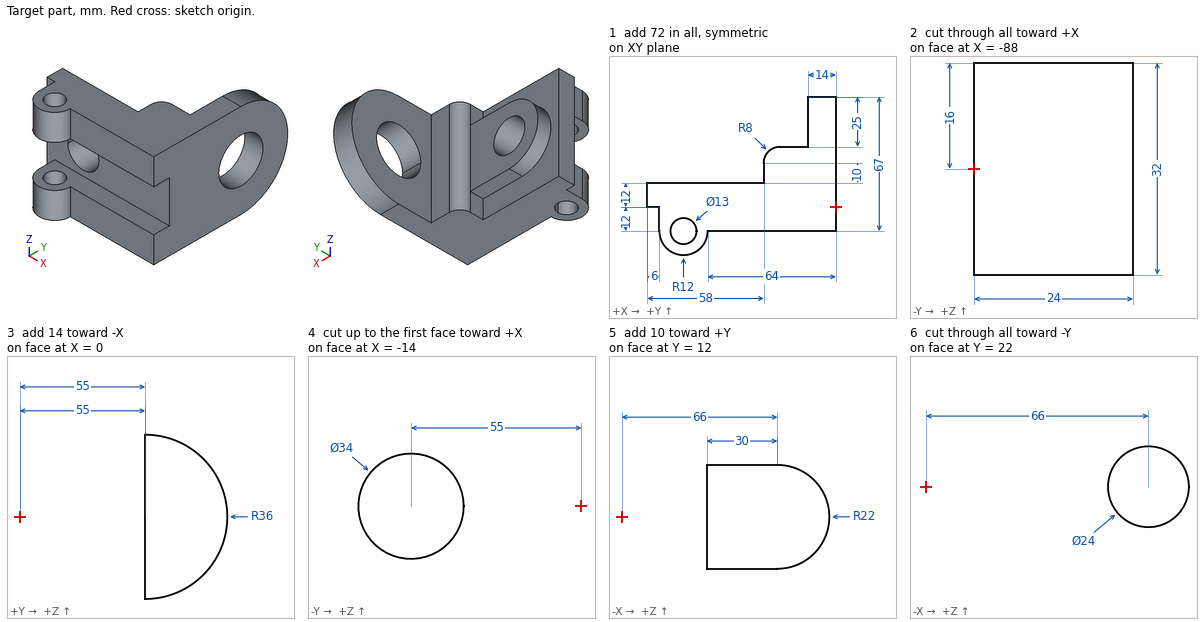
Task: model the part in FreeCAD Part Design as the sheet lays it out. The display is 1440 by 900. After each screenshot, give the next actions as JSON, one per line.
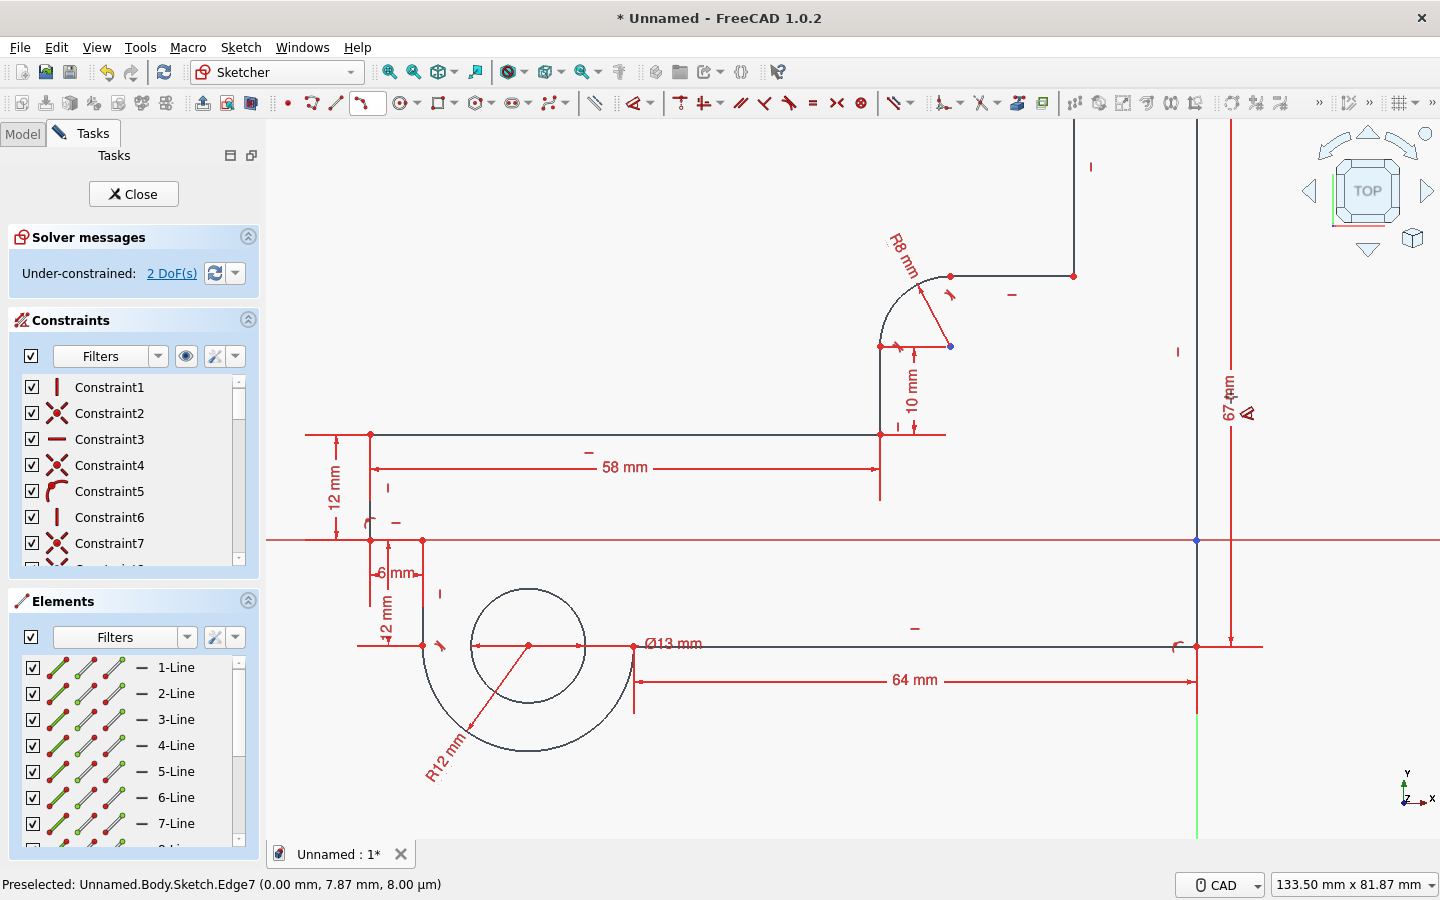
{"action": "scroll", "coordinate": [787, 632], "scroll_direction": "down", "scroll_amount": 2}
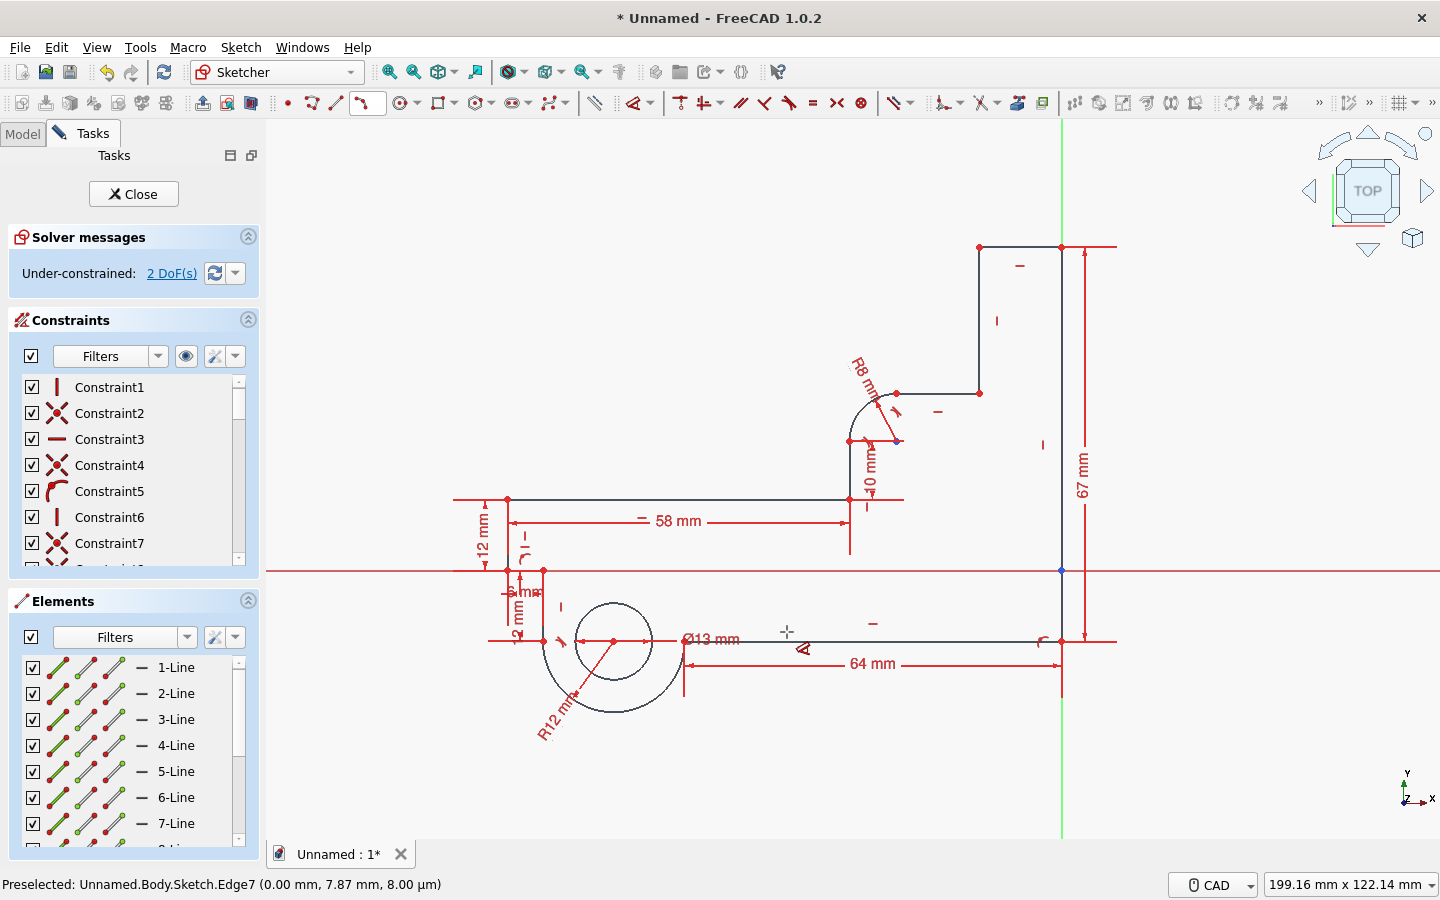
{"action": "left_click", "coordinate": [1037, 247]}
{"action": "left_click", "coordinate": [1021, 213]}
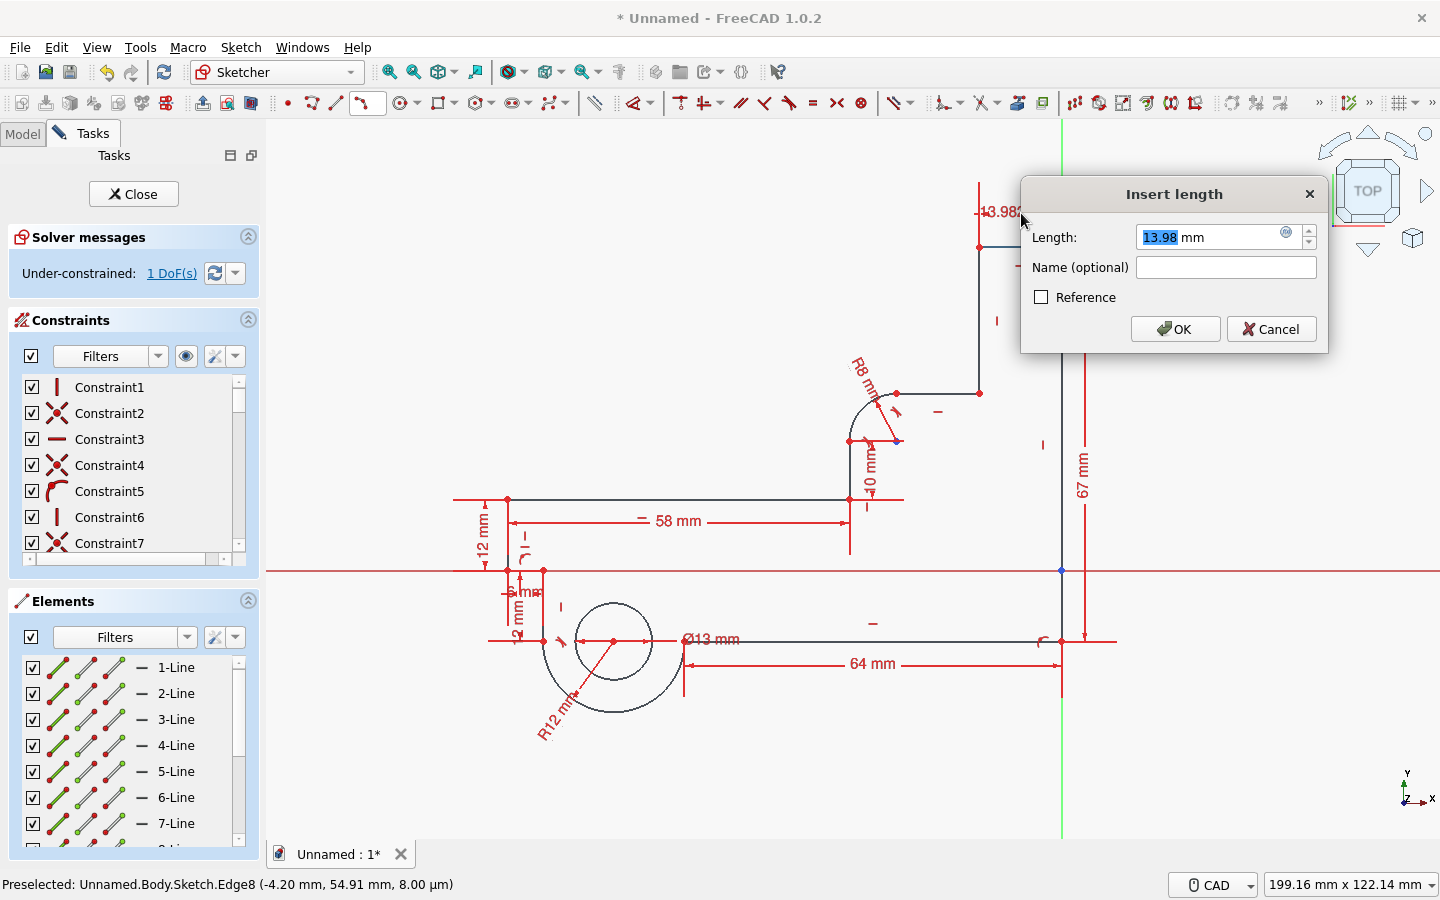
{"action": "type", "text": "14"}
{"action": "key", "text": "Return"}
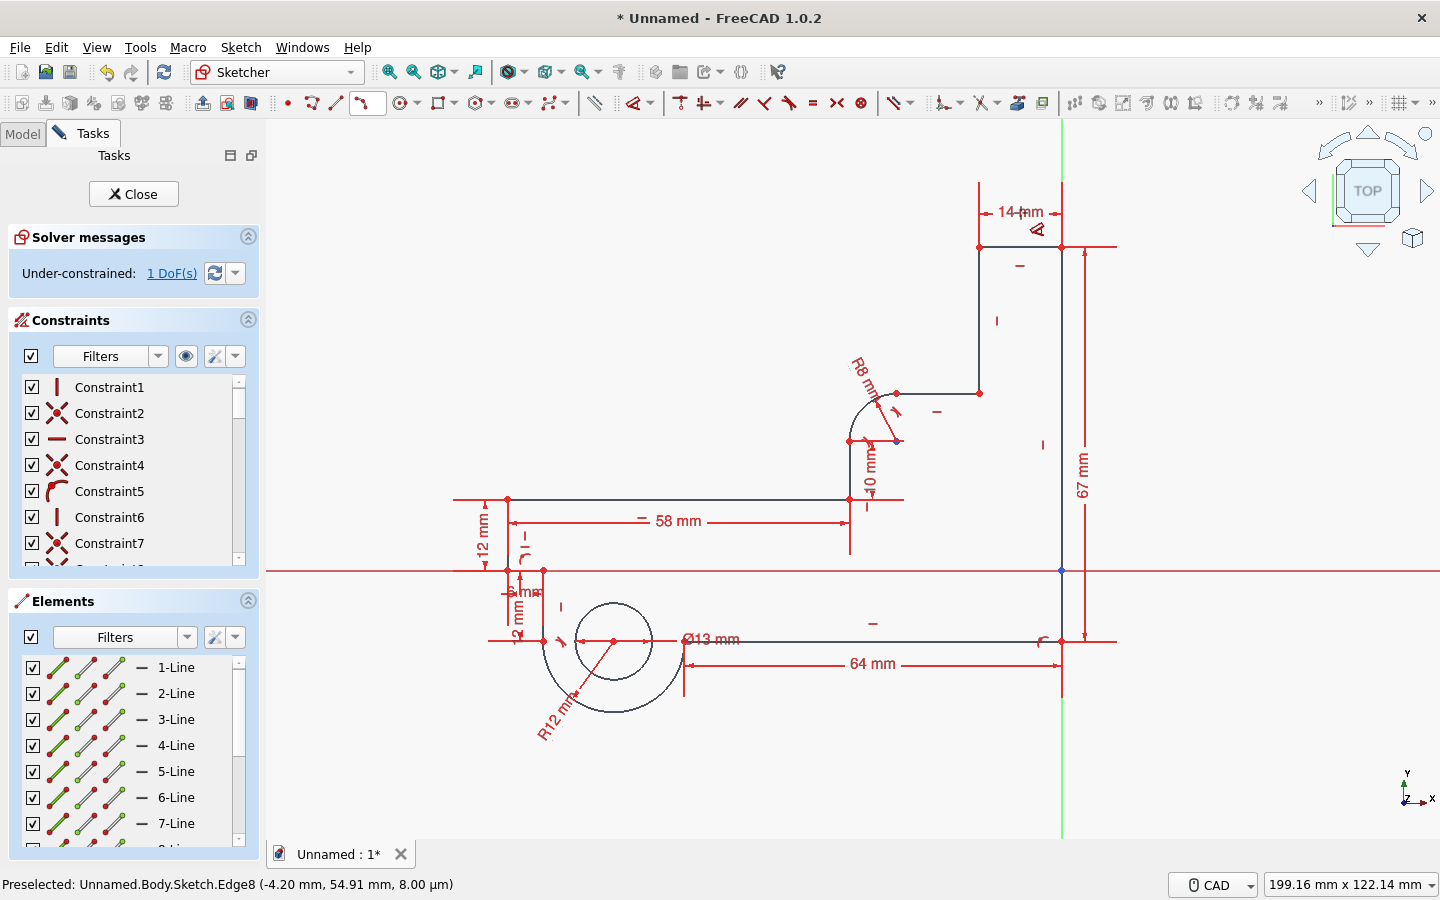
{"action": "left_click", "coordinate": [979, 291]}
{"action": "left_click", "coordinate": [1013, 320]}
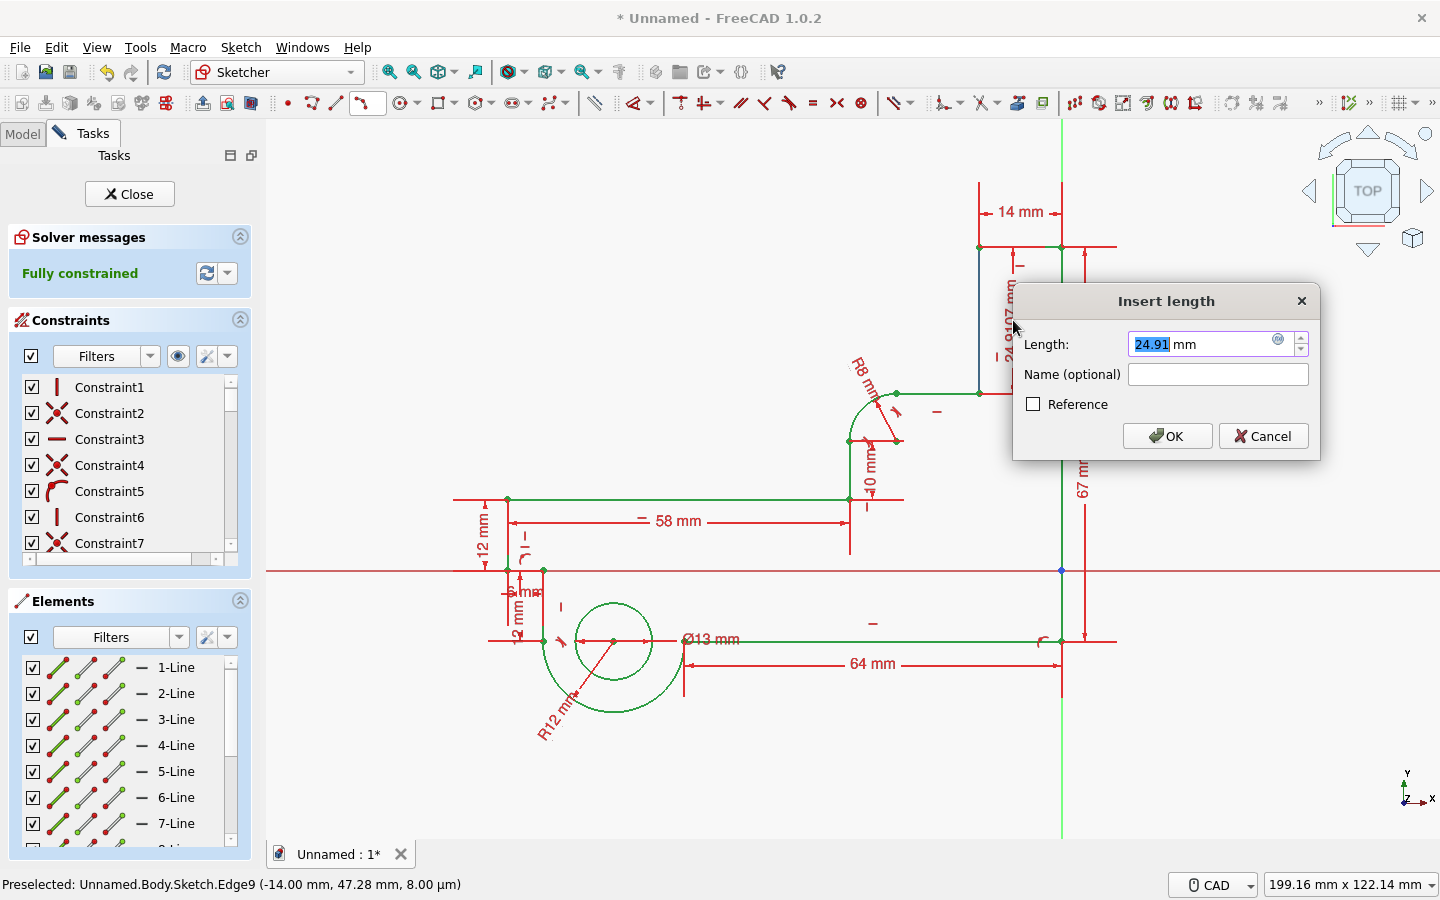
{"action": "type", "text": "25"}
{"action": "key", "text": "Return"}
{"action": "key", "text": "Escape"}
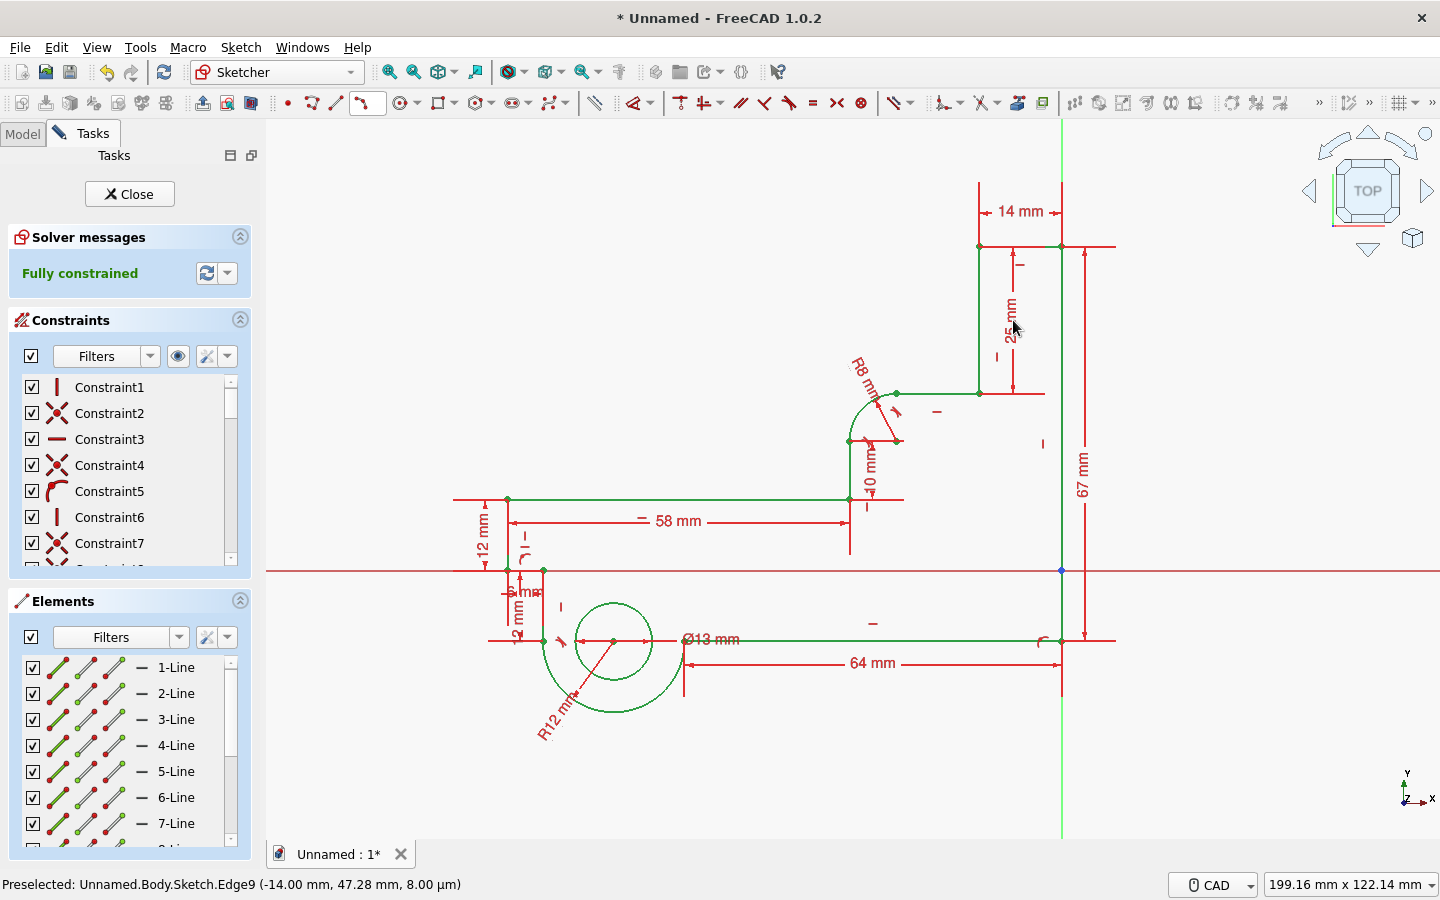
{"action": "left_click", "coordinate": [130, 194]}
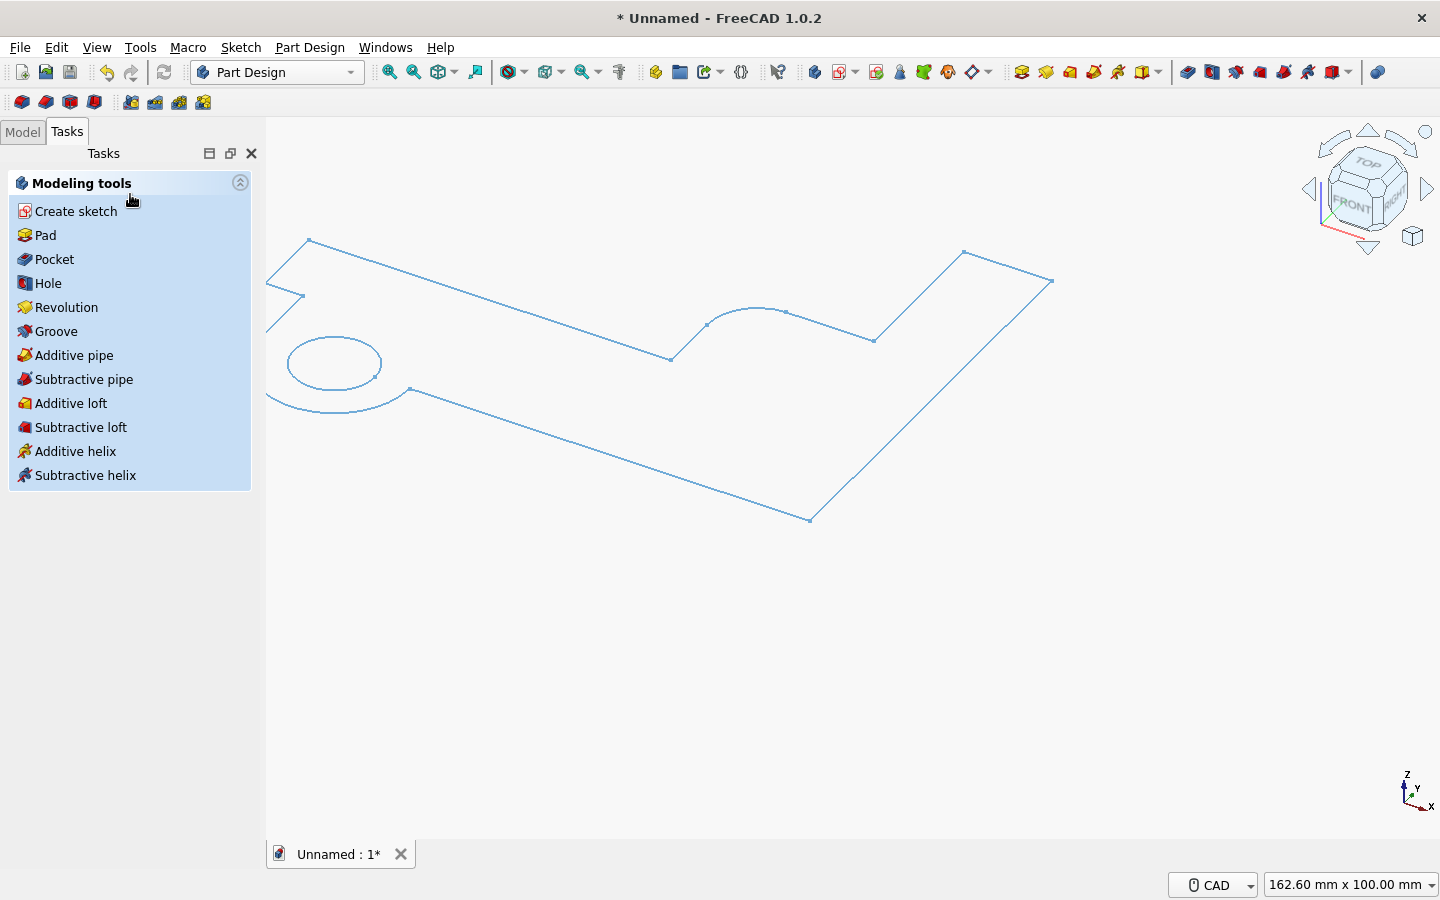
{"action": "left_click", "coordinate": [1022, 72]}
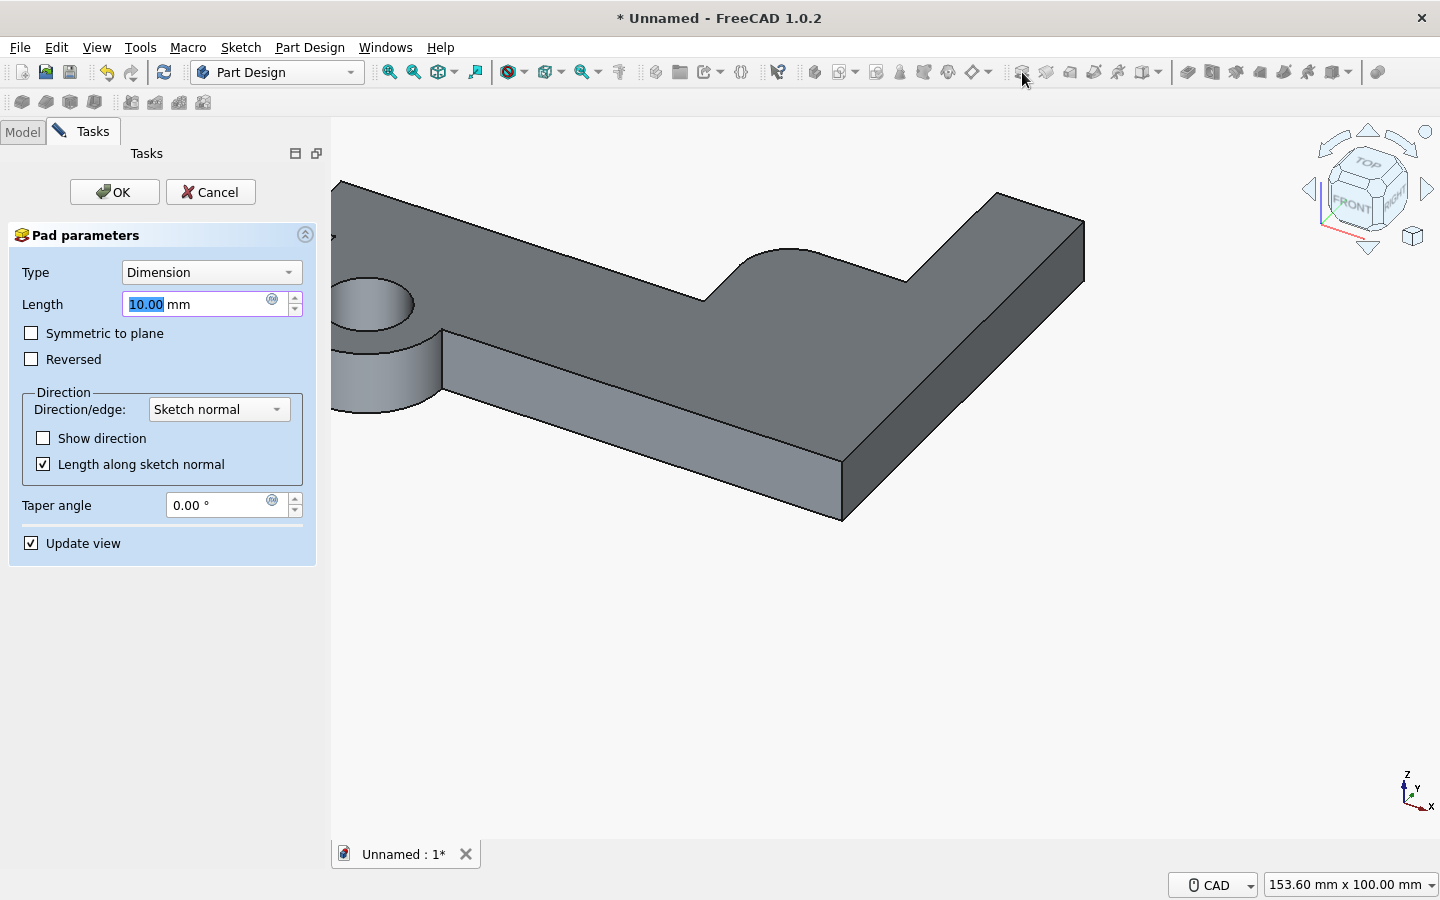
{"action": "type", "text": "72"}
{"action": "key", "text": "Tab"}